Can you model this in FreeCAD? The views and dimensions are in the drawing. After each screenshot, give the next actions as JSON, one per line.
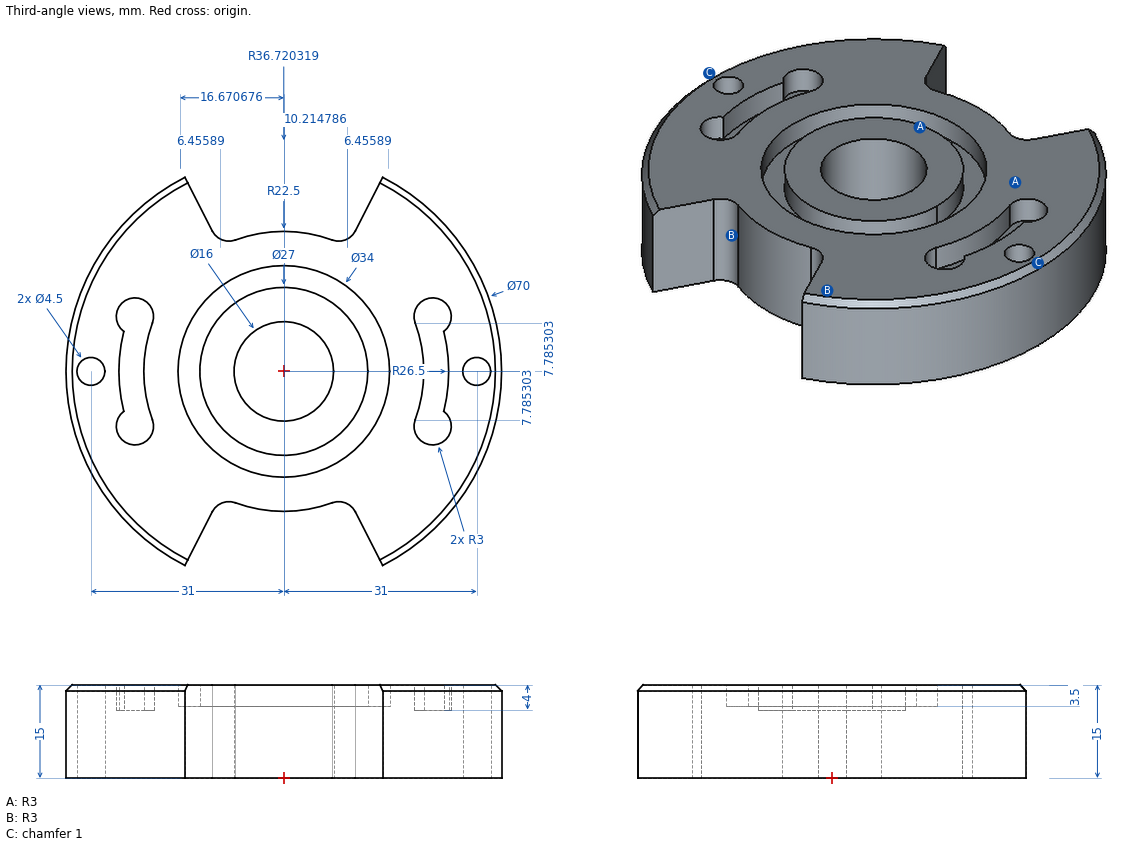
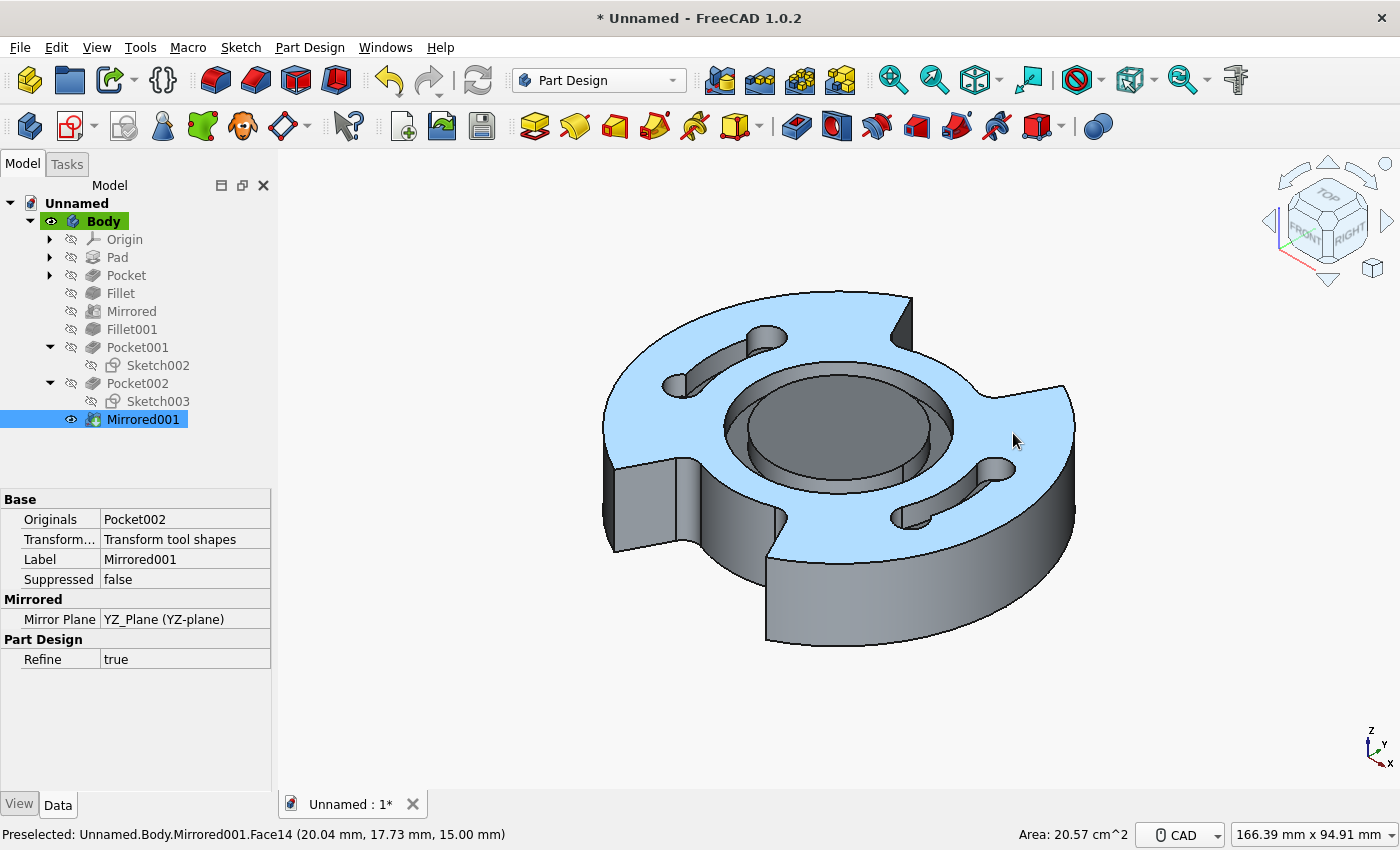
{"action": "left_click", "coordinate": [70, 126]}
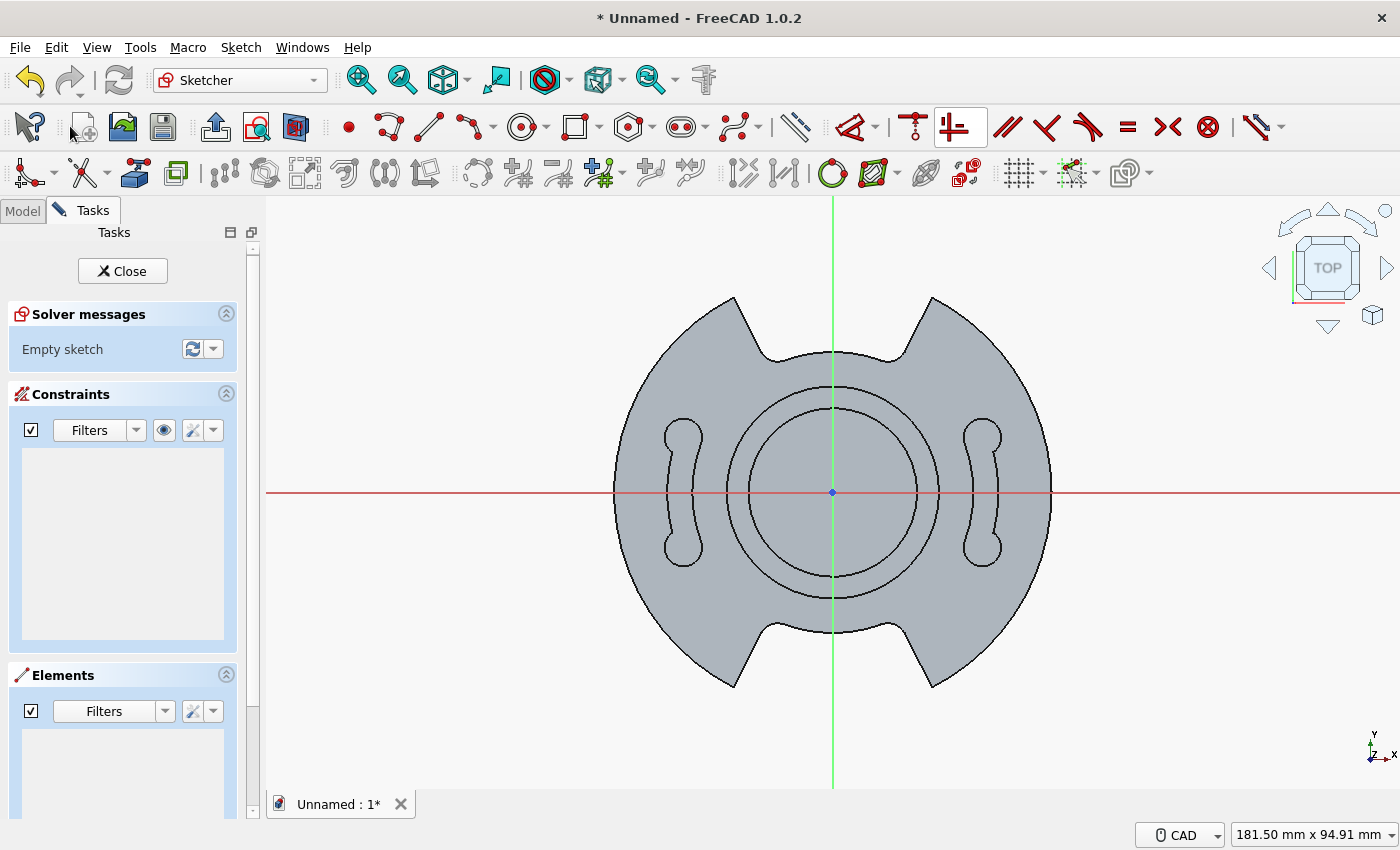
{"action": "scroll", "coordinate": [855, 493], "scroll_direction": "up", "scroll_amount": 7}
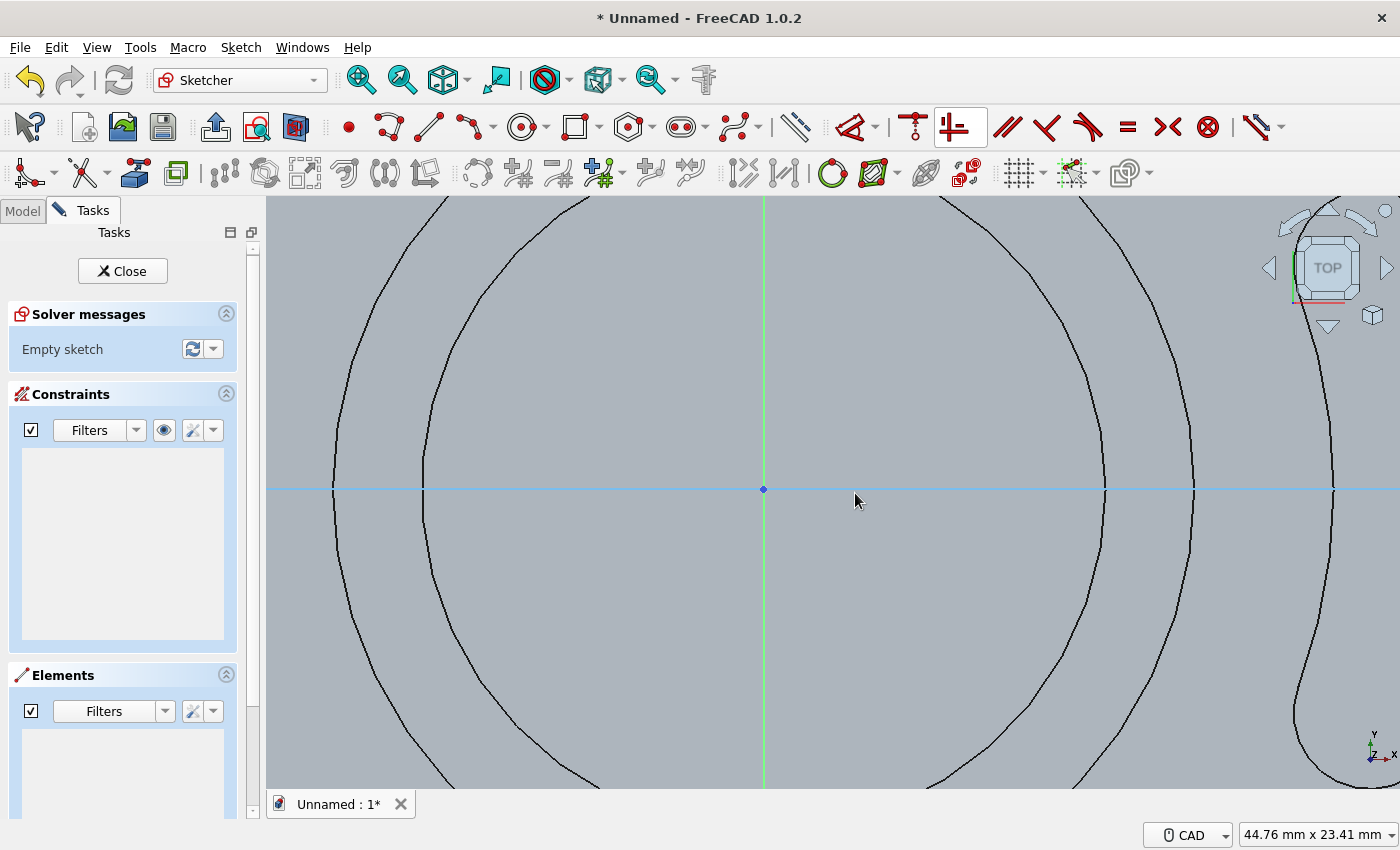
{"action": "left_click", "coordinate": [522, 128]}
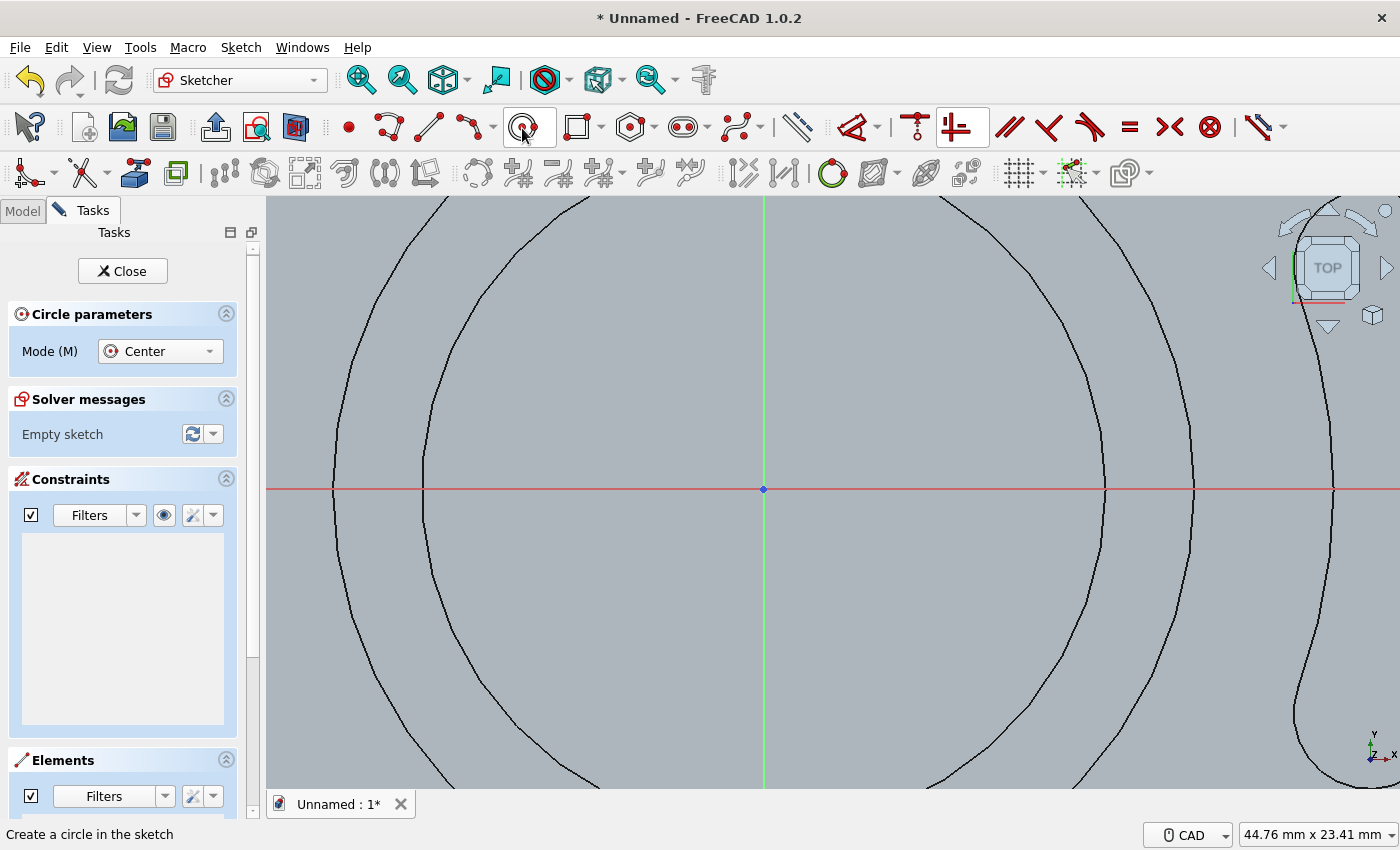
{"action": "left_click", "coordinate": [764, 489]}
{"action": "mouse_move", "coordinate": [907, 346]}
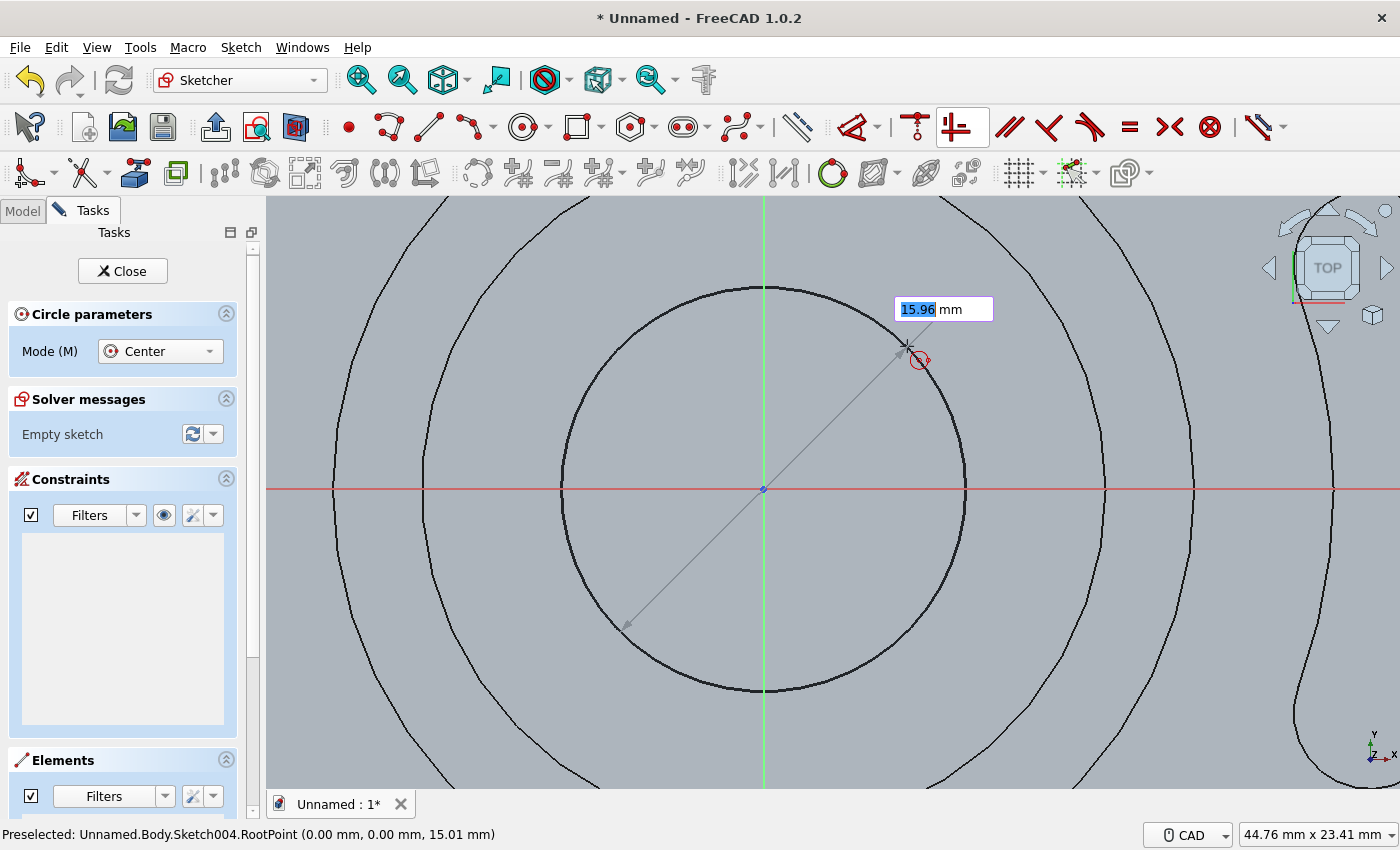
{"action": "type", "text": "16"}
{"action": "key", "text": "Return"}
{"action": "key", "text": "Escape"}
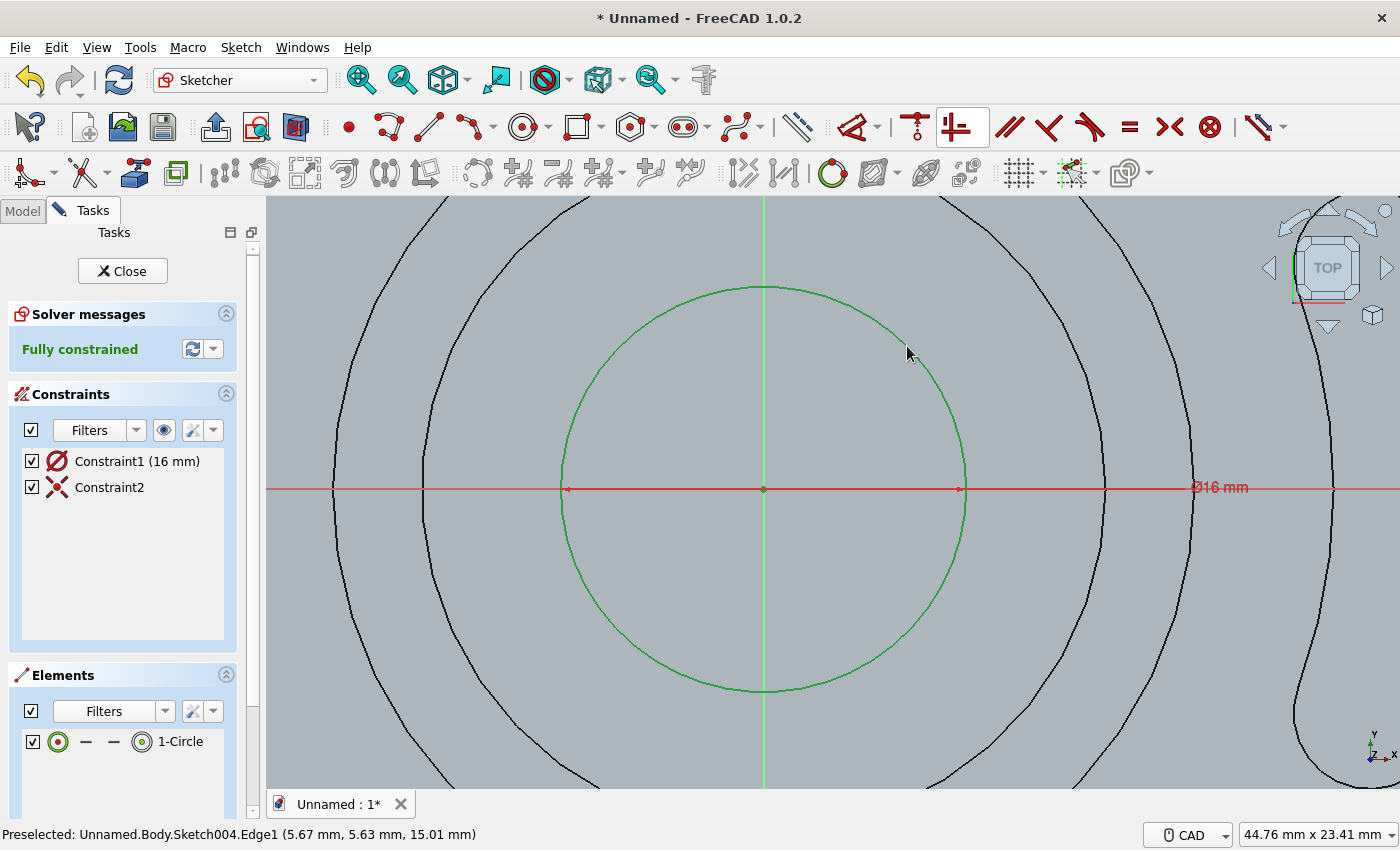
{"action": "left_click", "coordinate": [123, 271]}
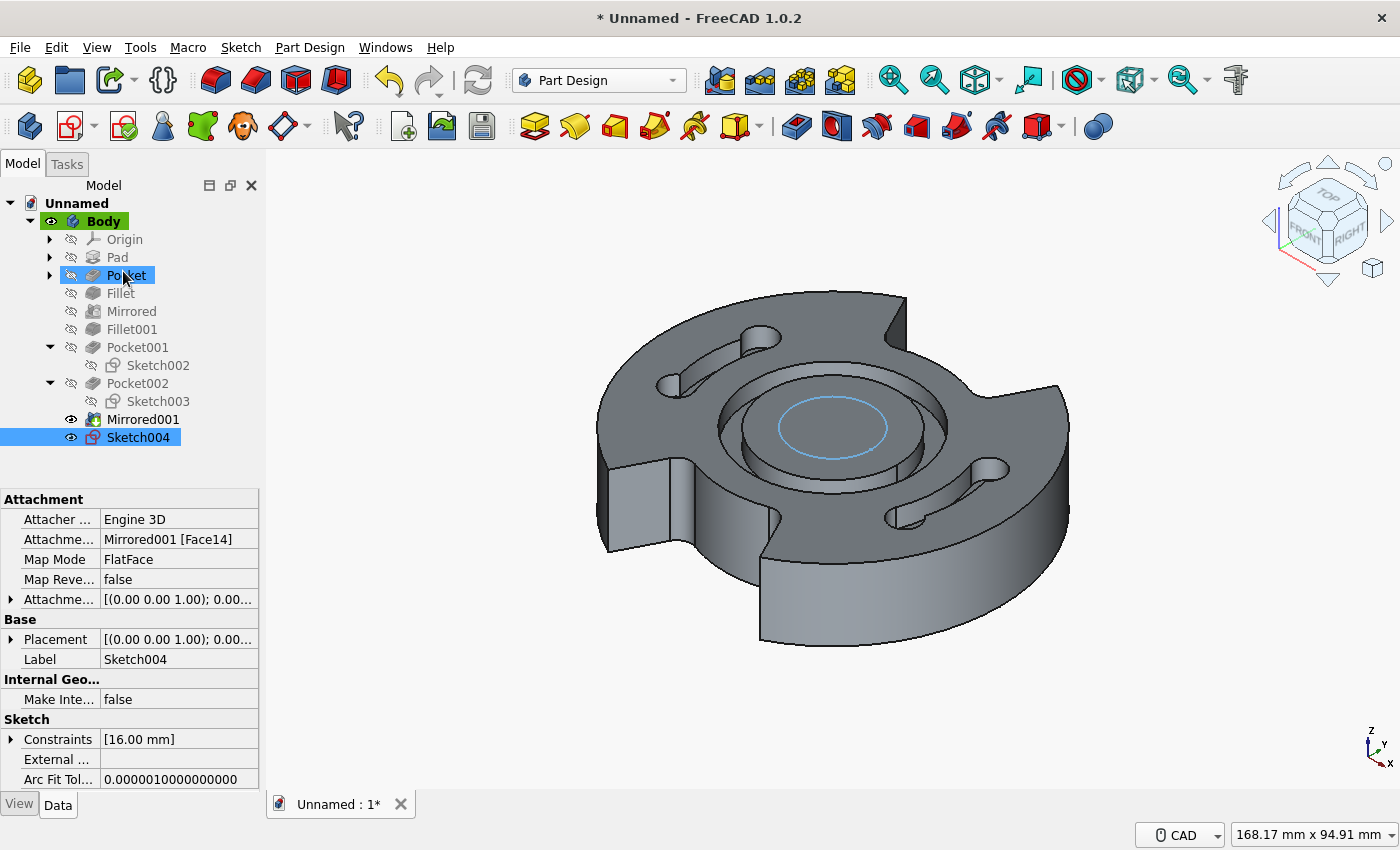
{"action": "left_click", "coordinate": [798, 126]}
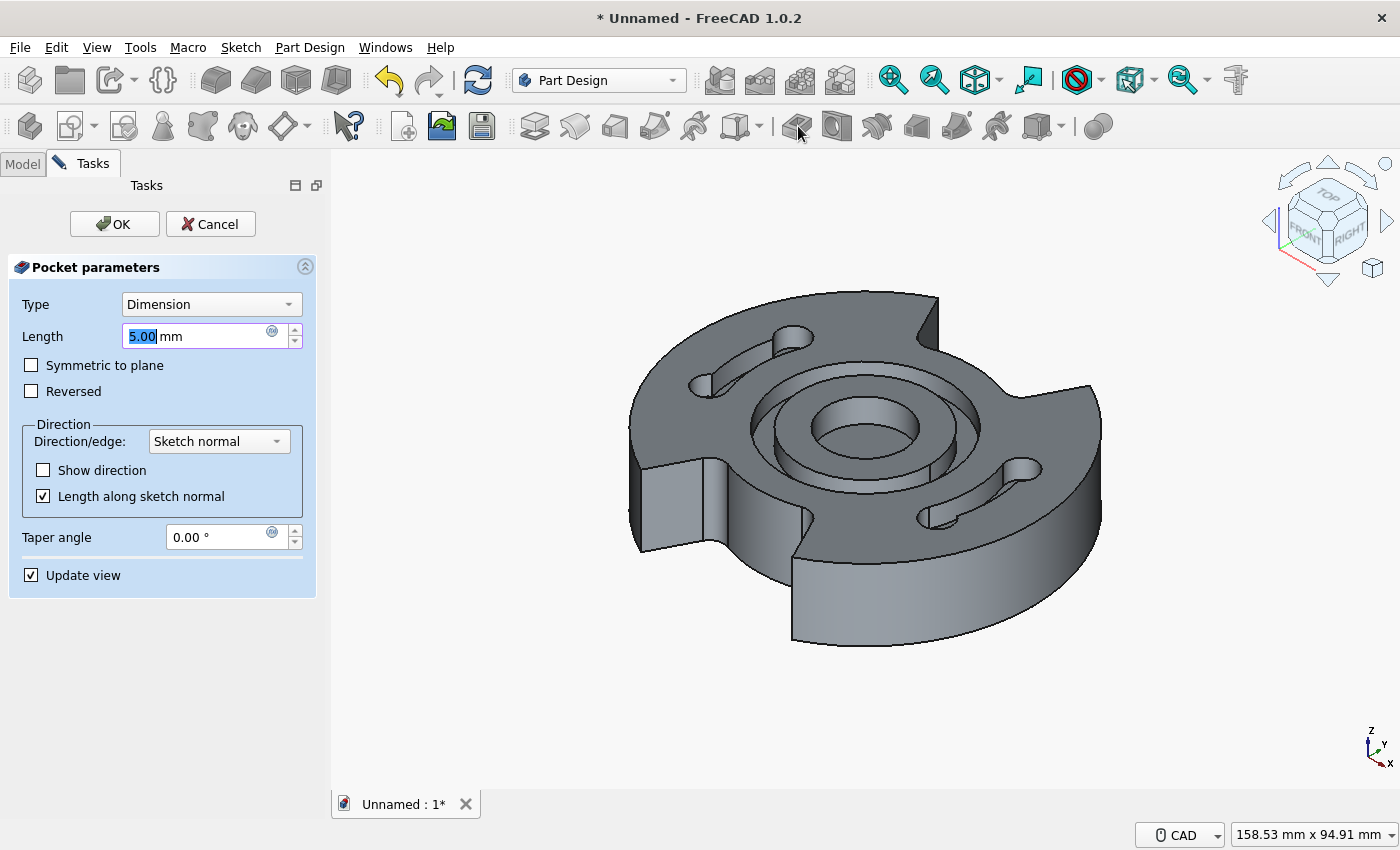
{"action": "left_click", "coordinate": [212, 304]}